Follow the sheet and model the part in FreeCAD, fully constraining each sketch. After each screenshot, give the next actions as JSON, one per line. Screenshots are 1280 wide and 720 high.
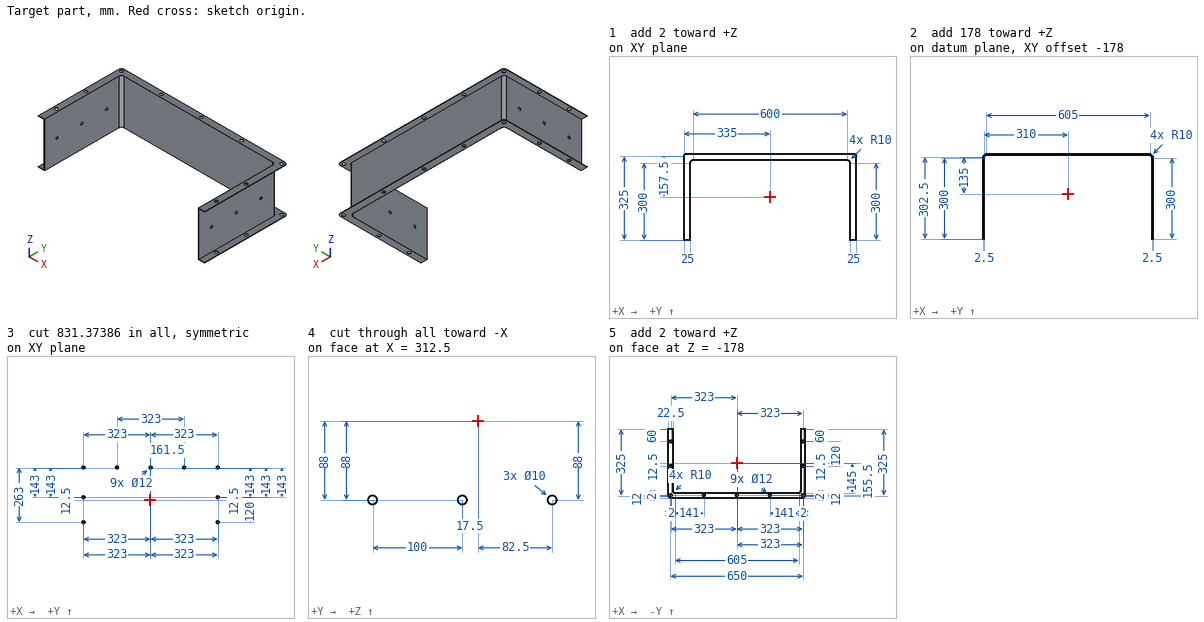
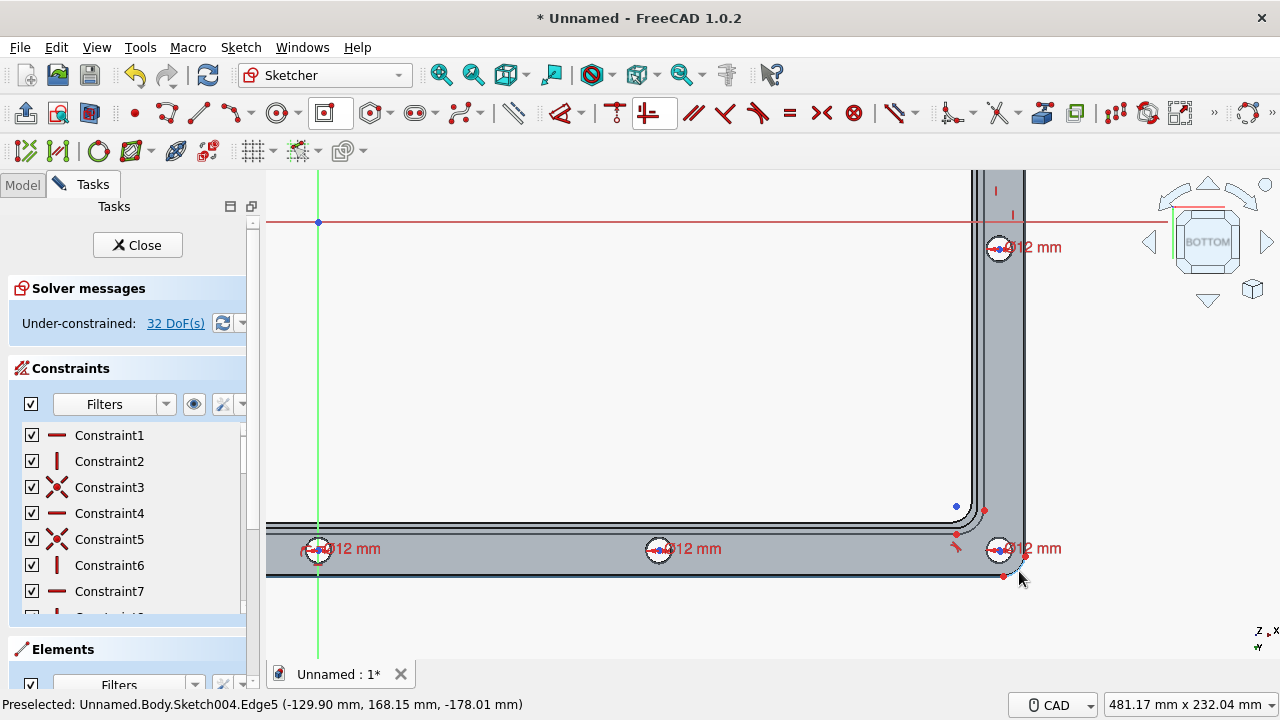
{"action": "left_click", "coordinate": [1018, 570]}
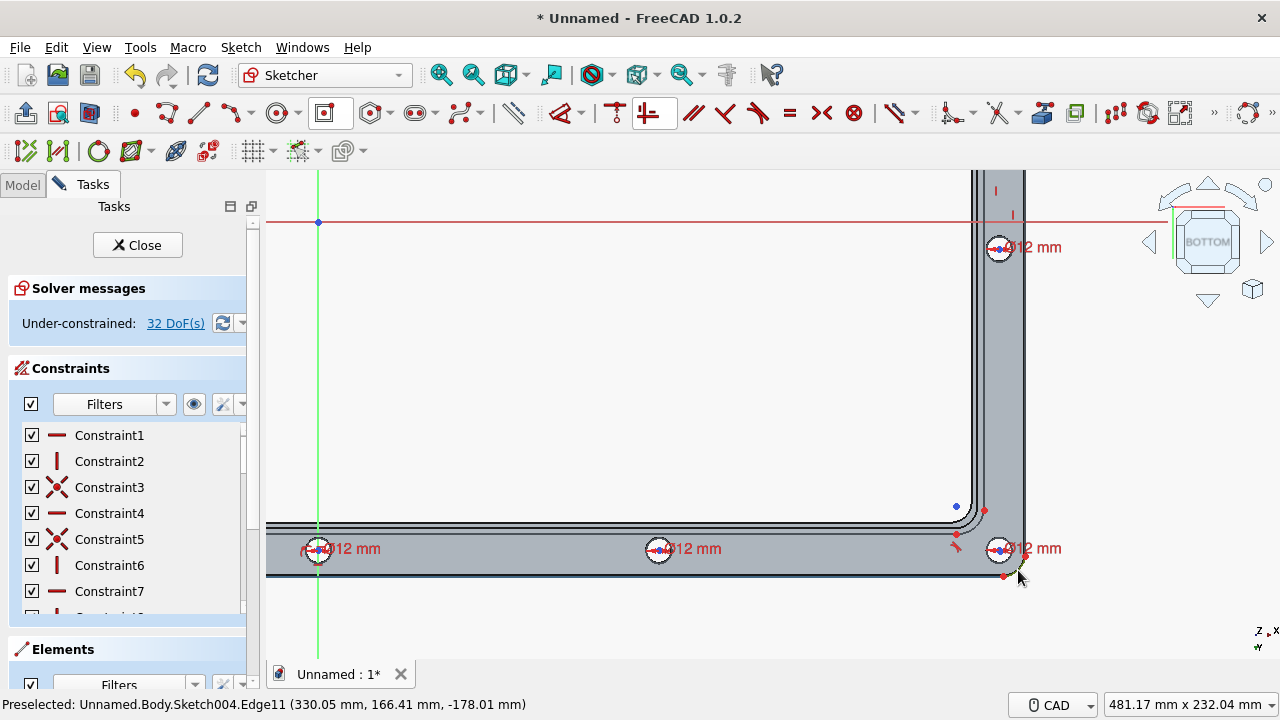
{"action": "key", "text": "t"}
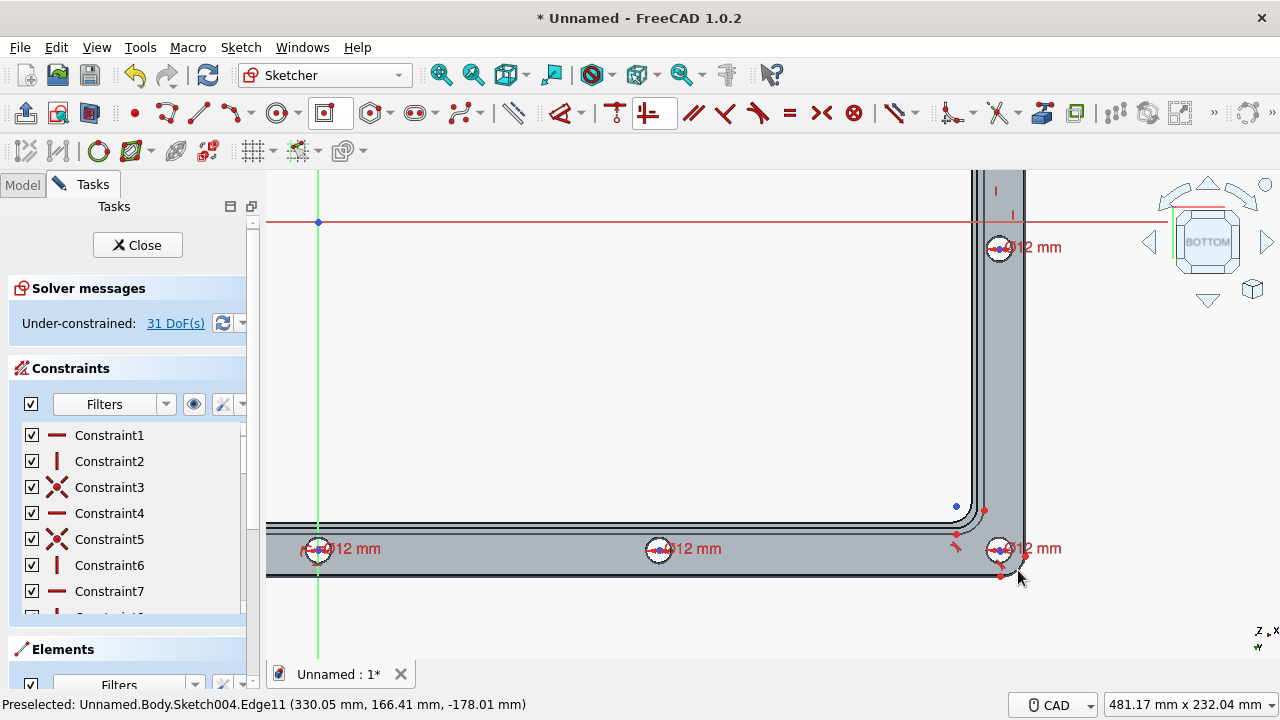
{"action": "left_click", "coordinate": [1025, 351]}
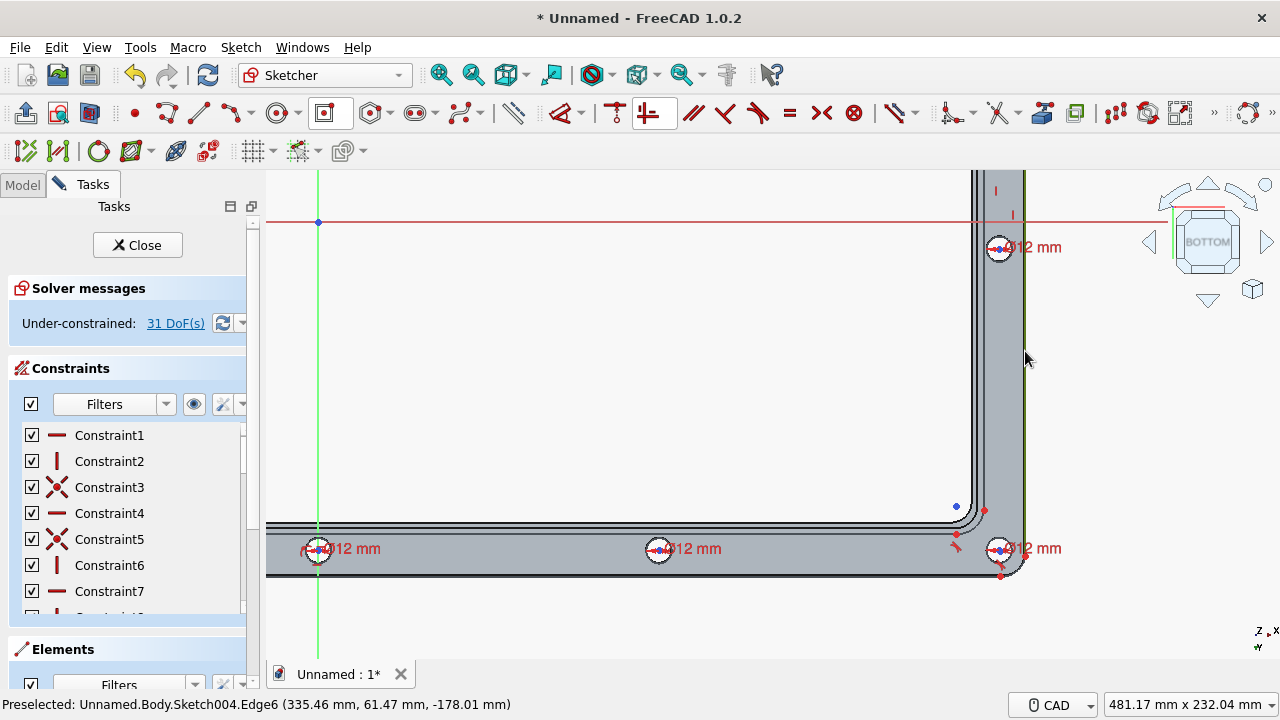
{"action": "scroll", "coordinate": [1011, 575], "scroll_direction": "up", "scroll_amount": 2}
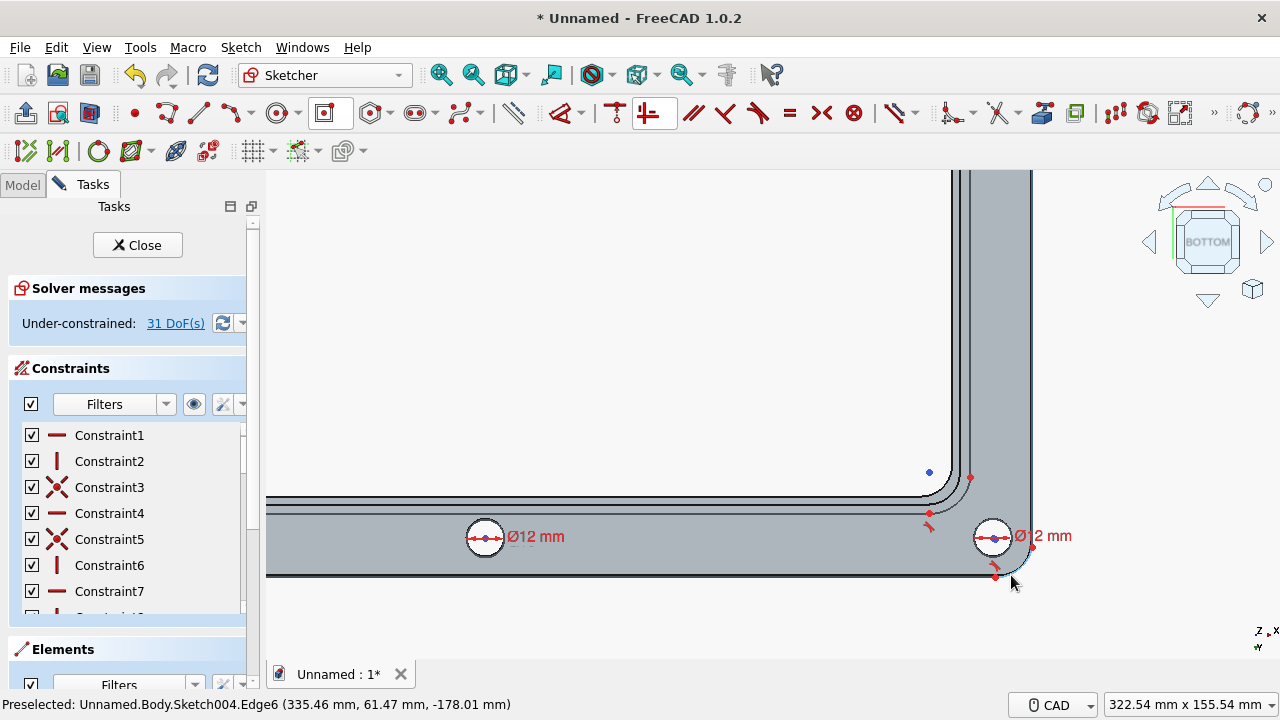
{"action": "left_click", "coordinate": [1010, 574]}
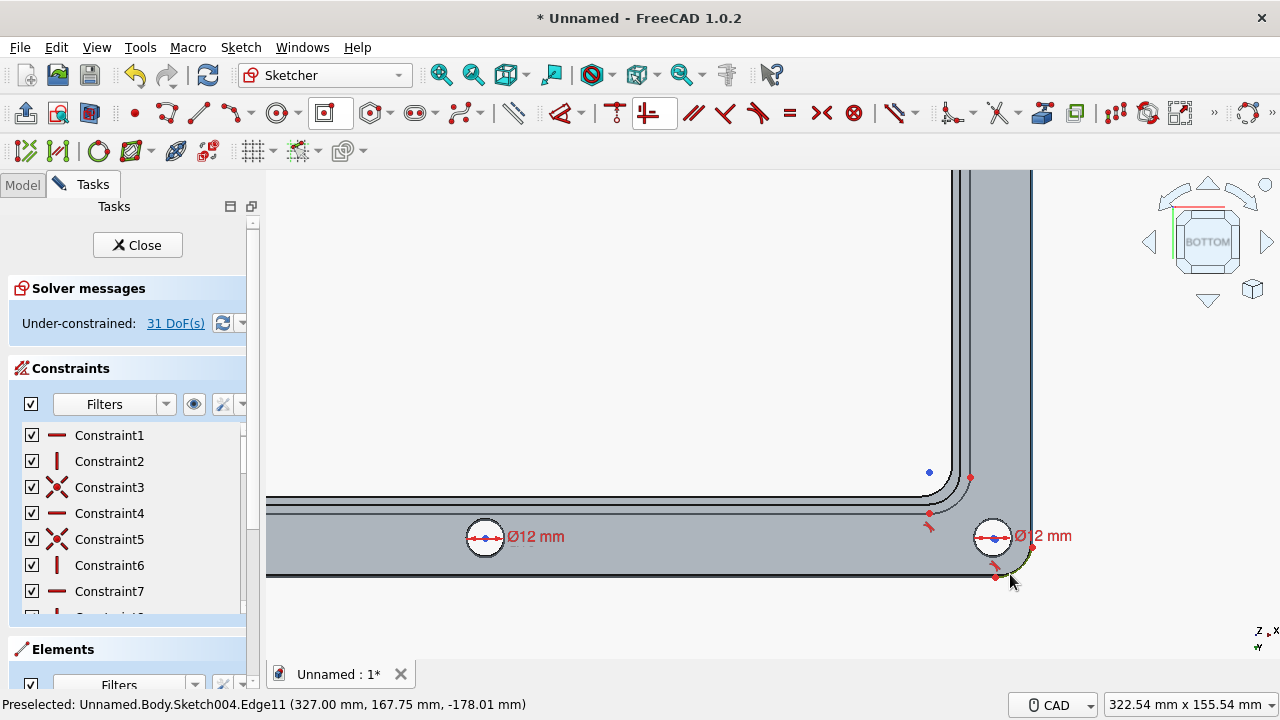
{"action": "left_click", "coordinate": [758, 114]}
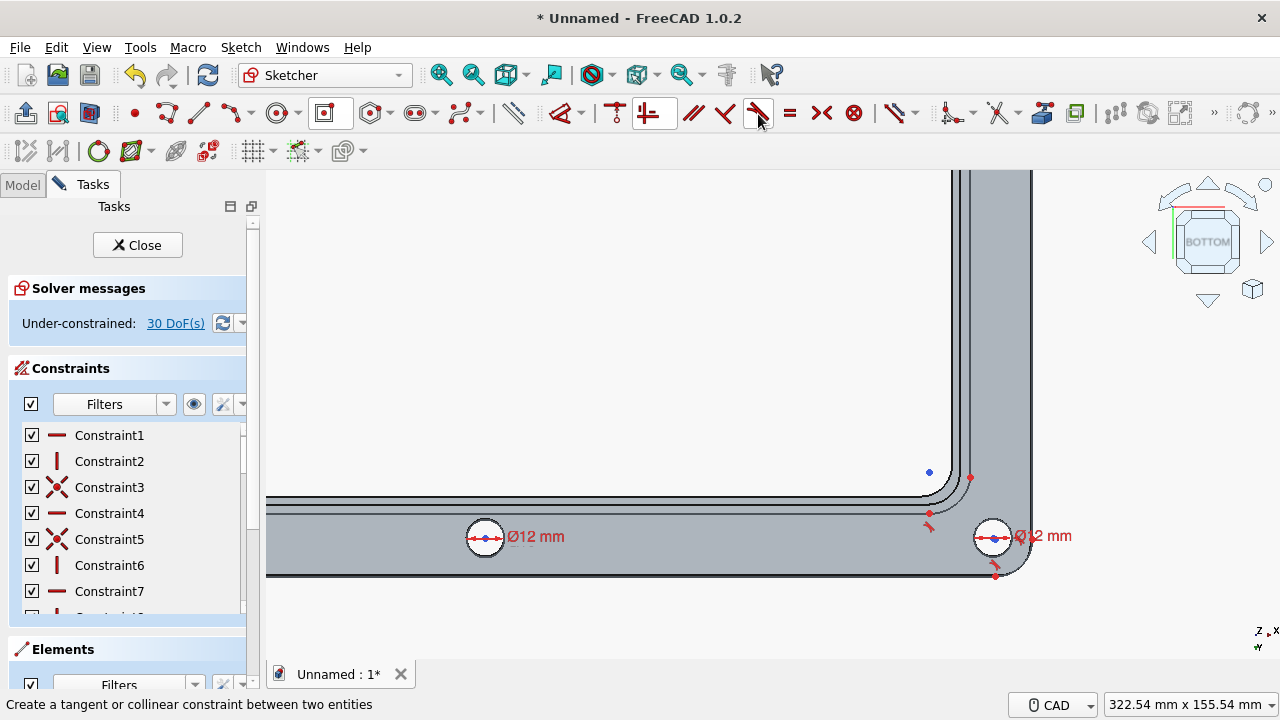
{"action": "left_click", "coordinate": [970, 287]}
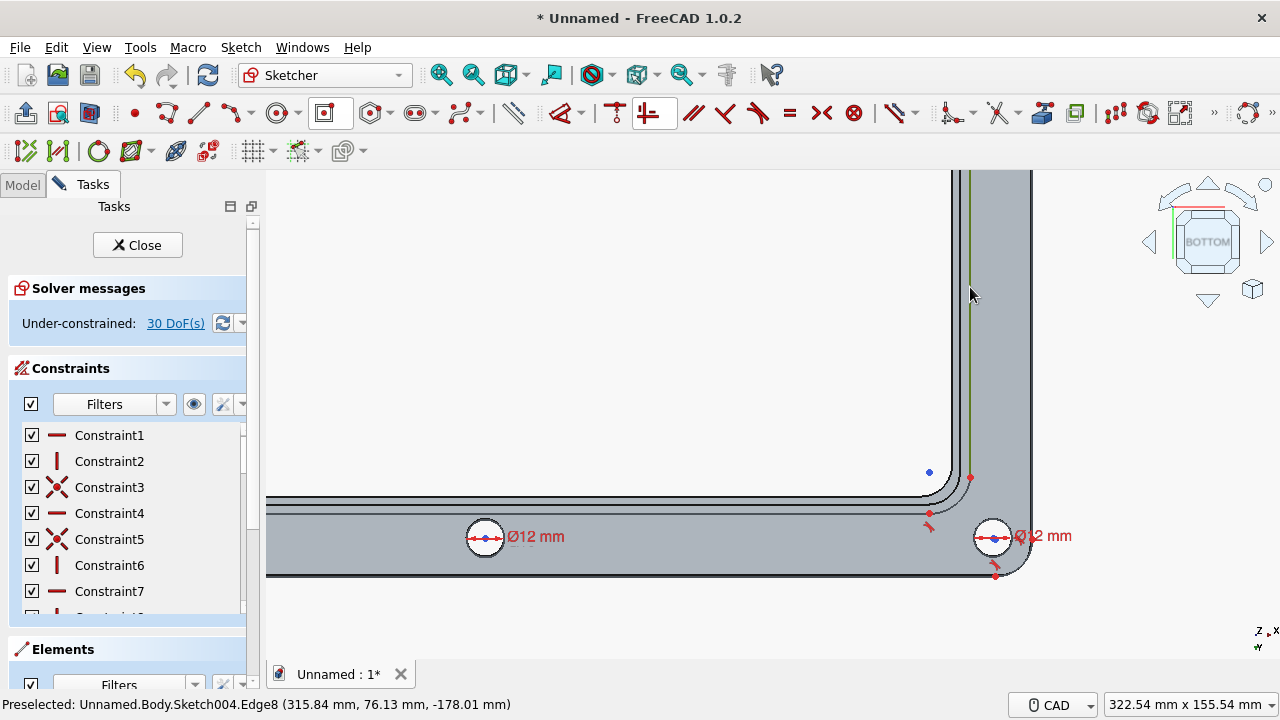
{"action": "left_click", "coordinate": [947, 510]}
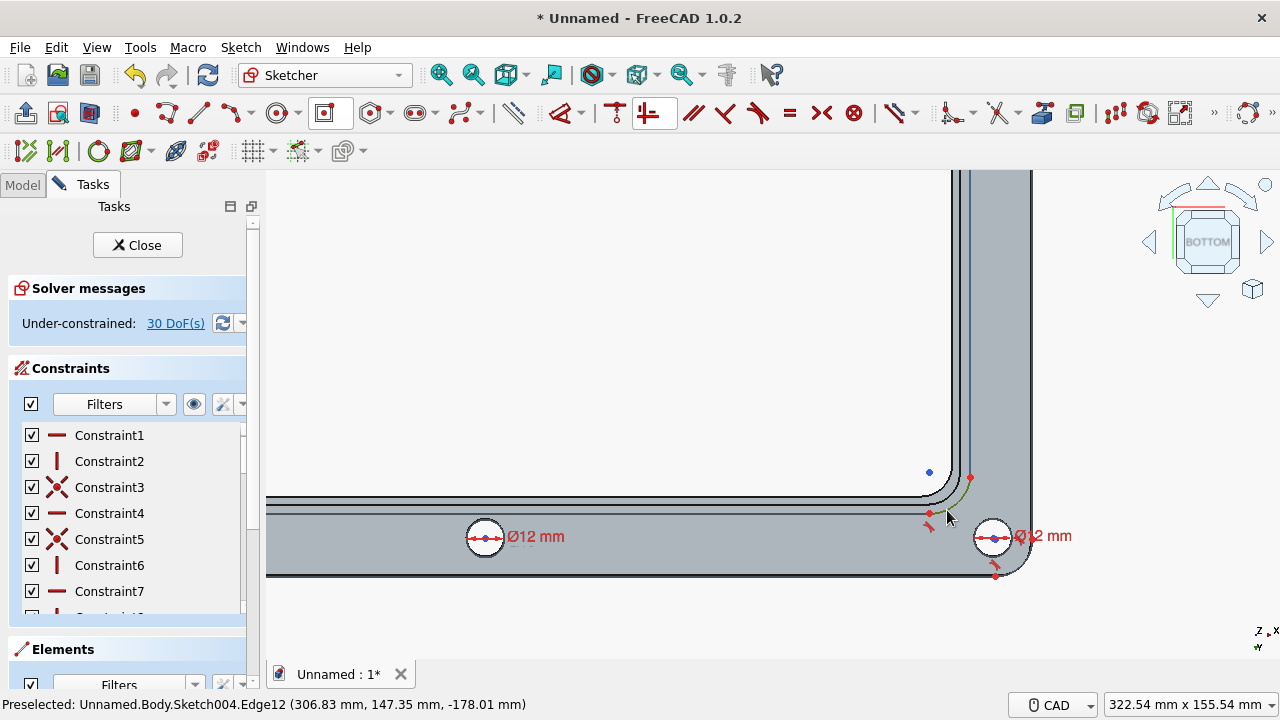
{"action": "left_click", "coordinate": [758, 114]}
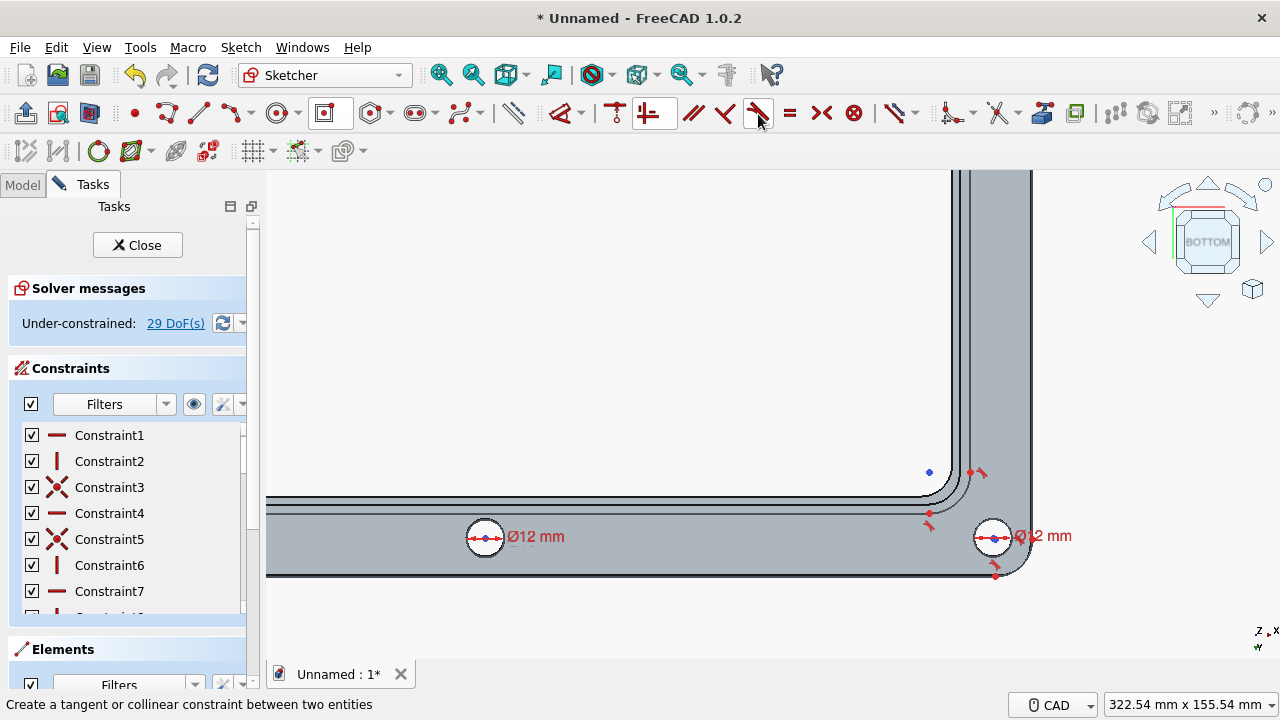
{"action": "scroll", "coordinate": [1018, 572], "scroll_direction": "down", "scroll_amount": 6}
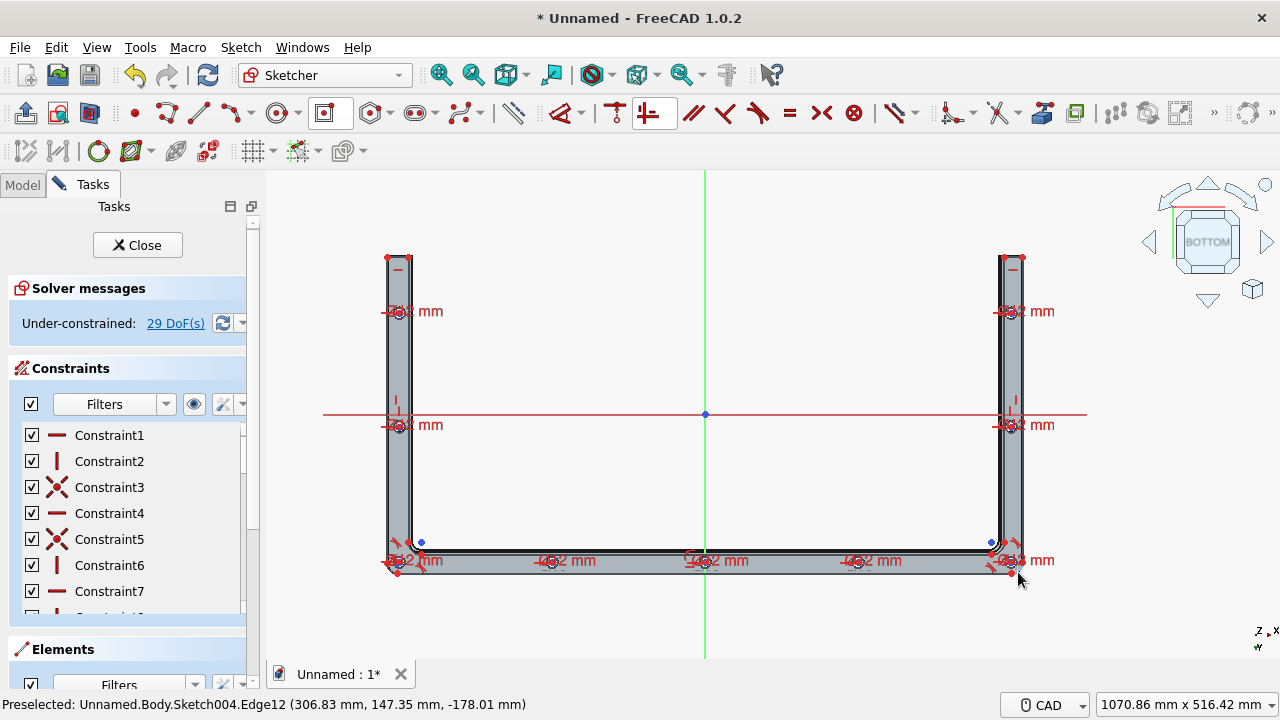
{"action": "scroll", "coordinate": [410, 548], "scroll_direction": "up", "scroll_amount": 5}